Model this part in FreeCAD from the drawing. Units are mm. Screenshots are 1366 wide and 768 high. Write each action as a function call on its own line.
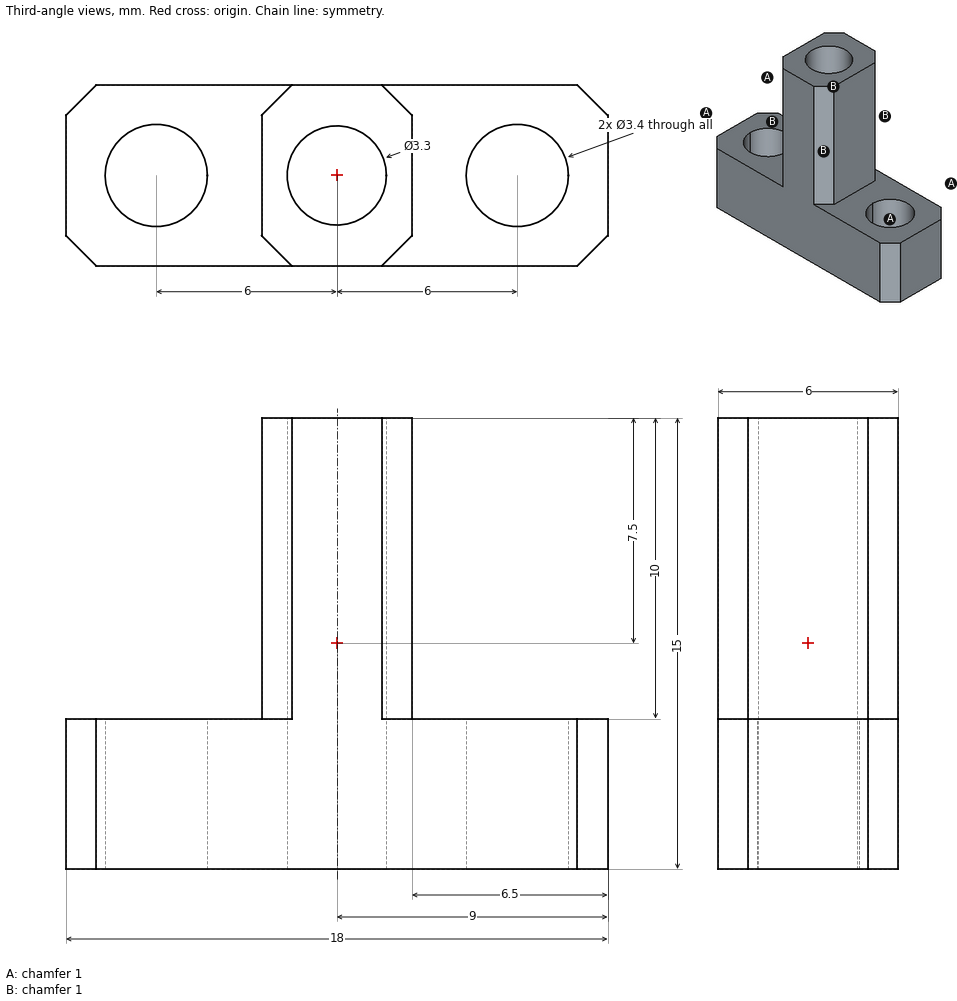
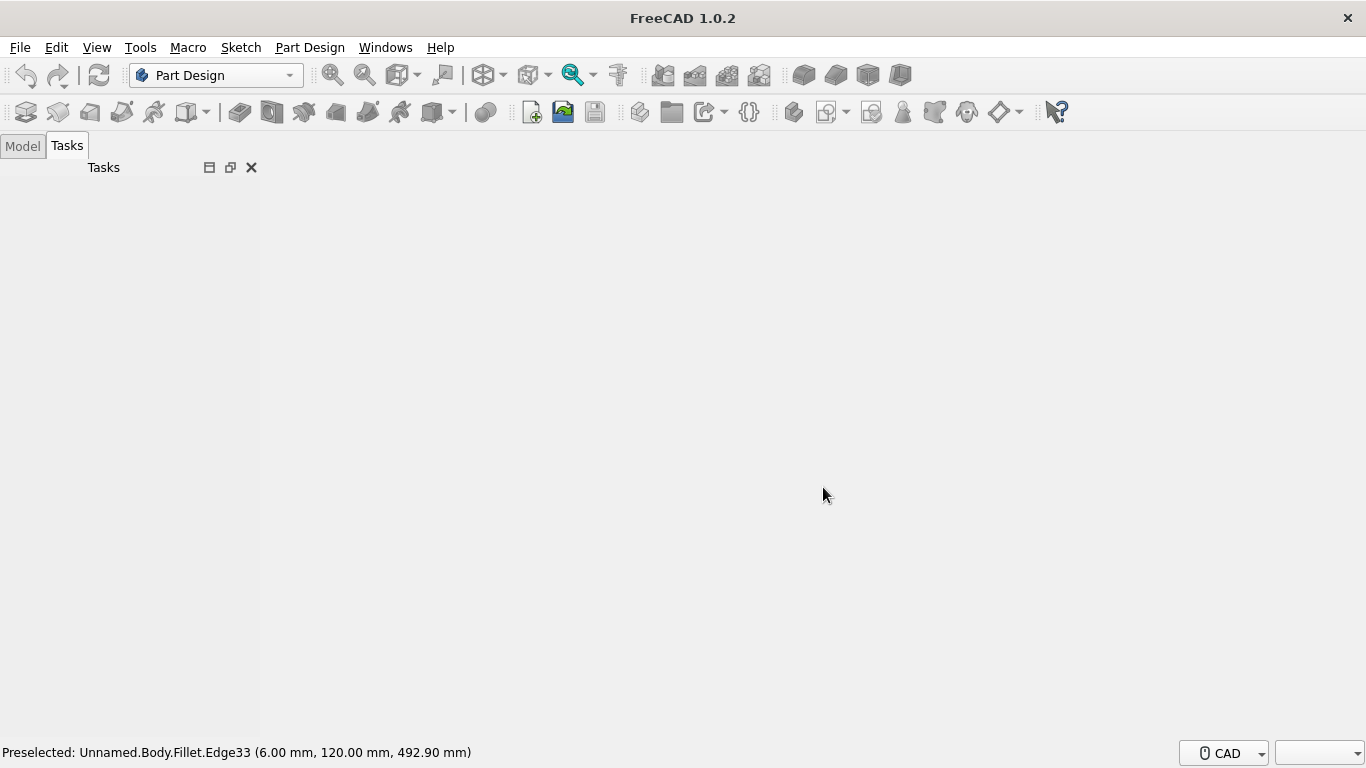
click(532, 112)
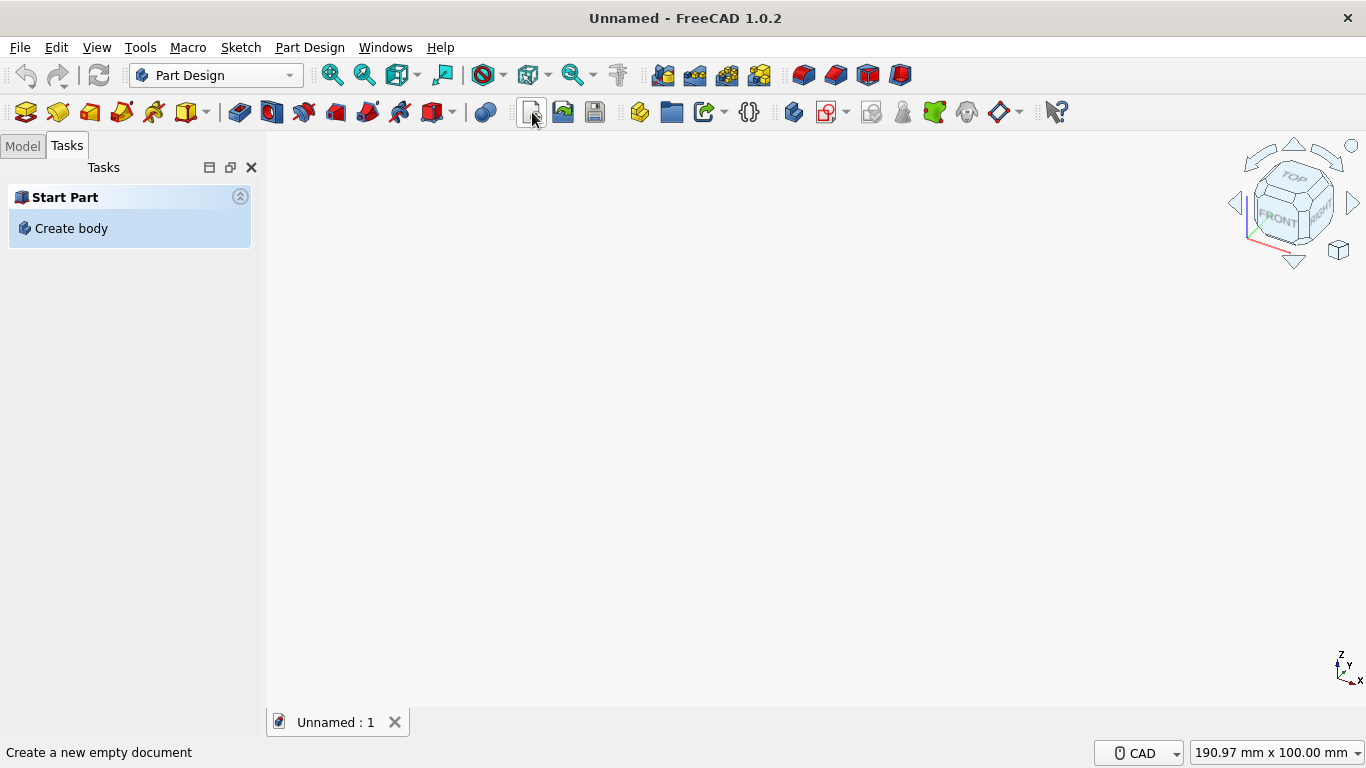
click(826, 112)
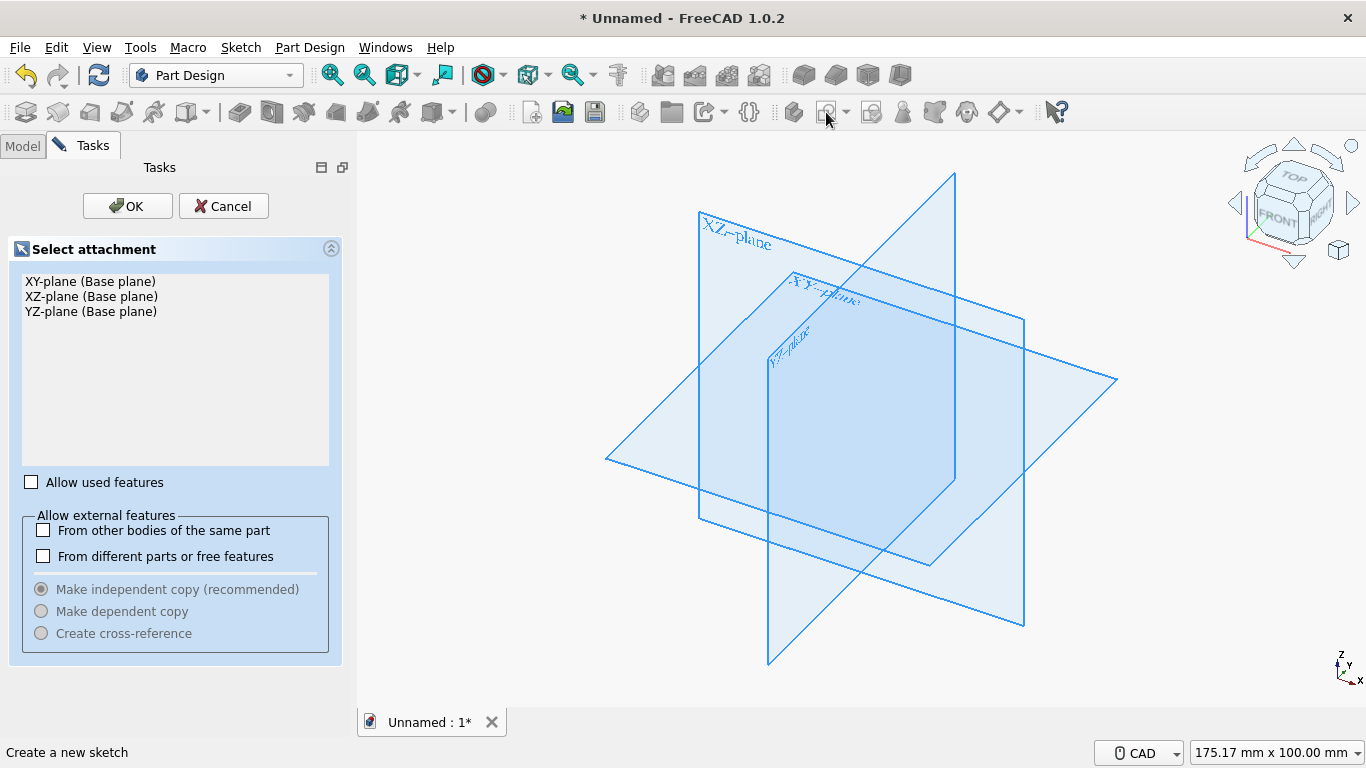
click(82, 296)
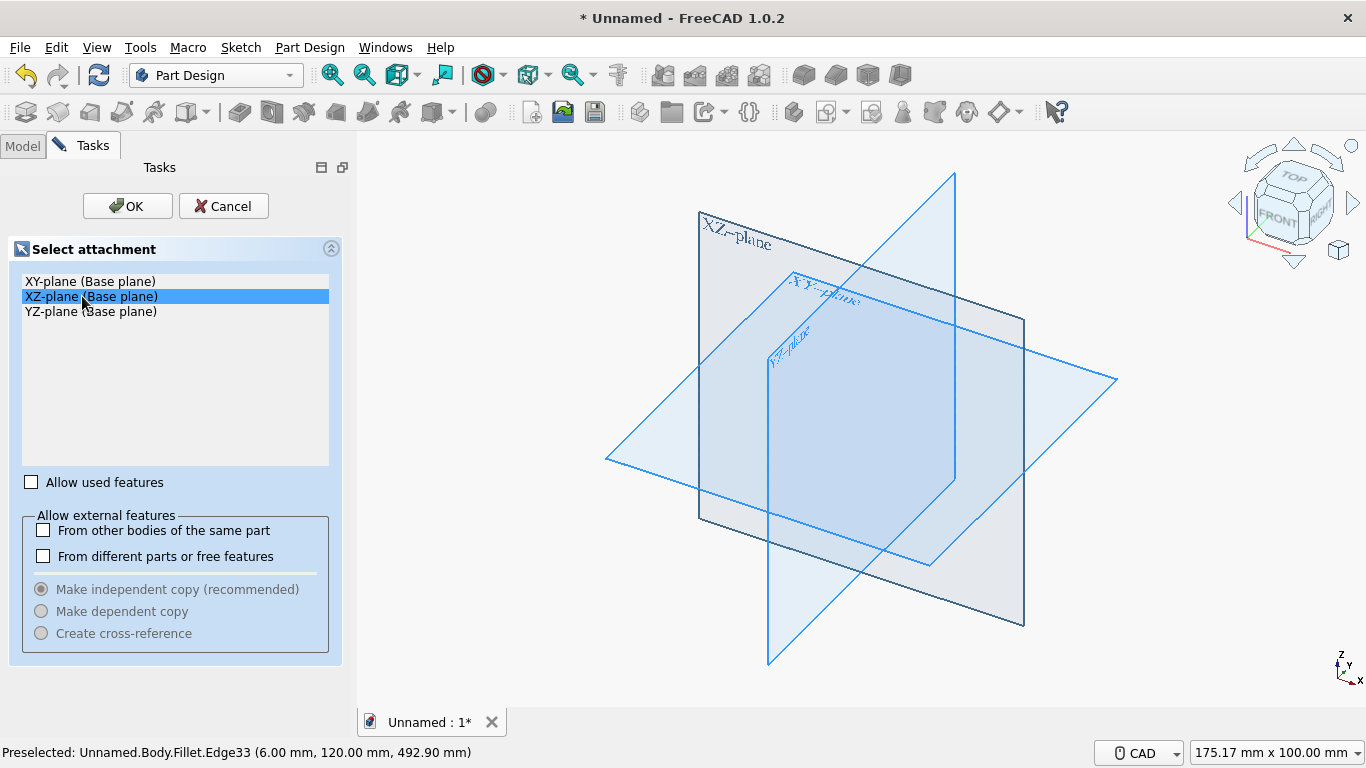
click(128, 206)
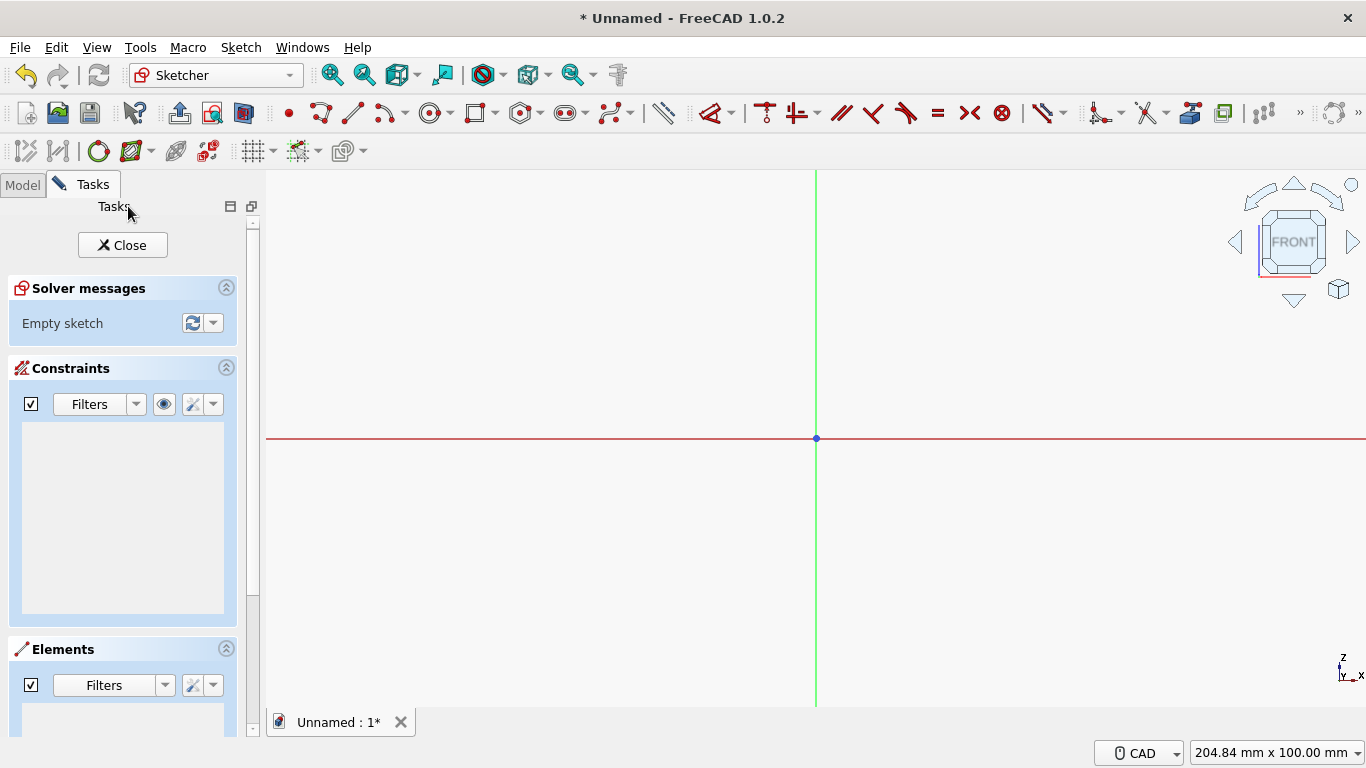
scroll(838, 438, up, 7)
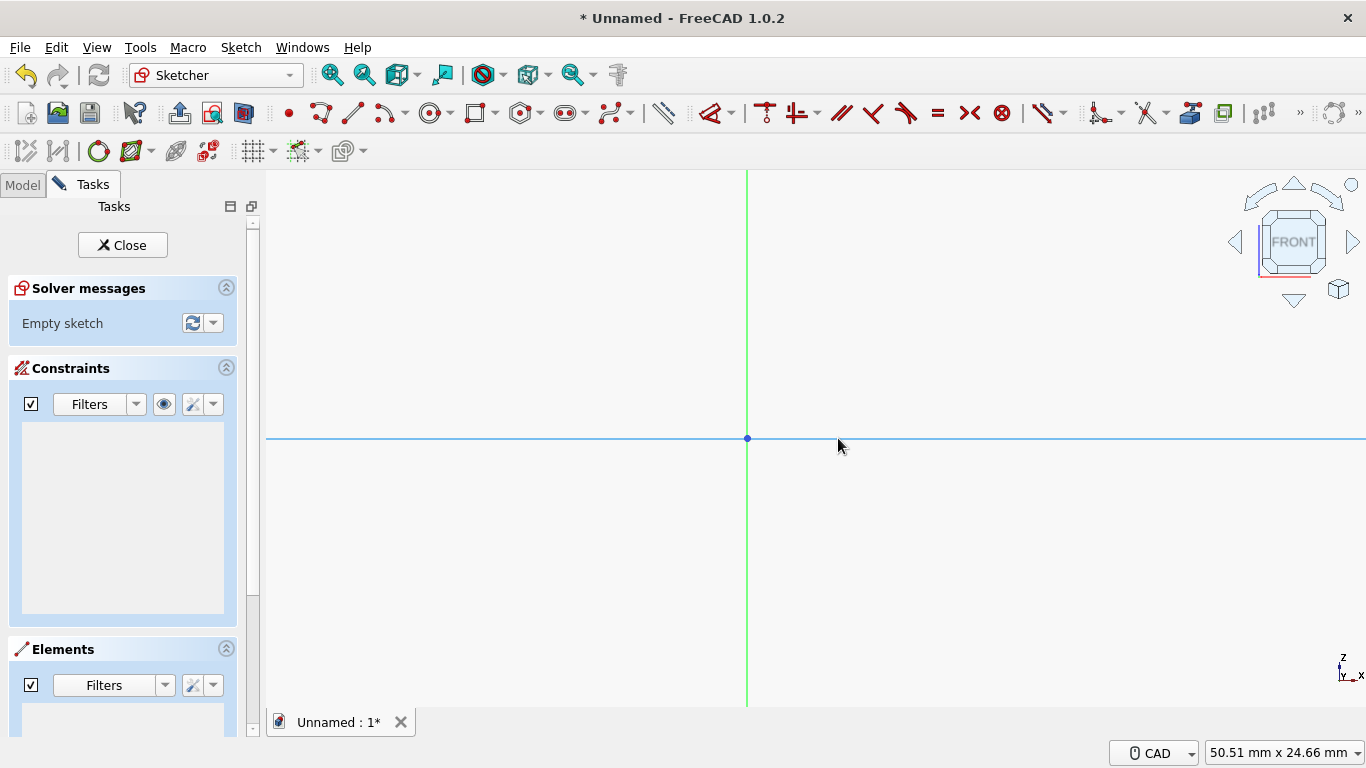
key(g)
key(v)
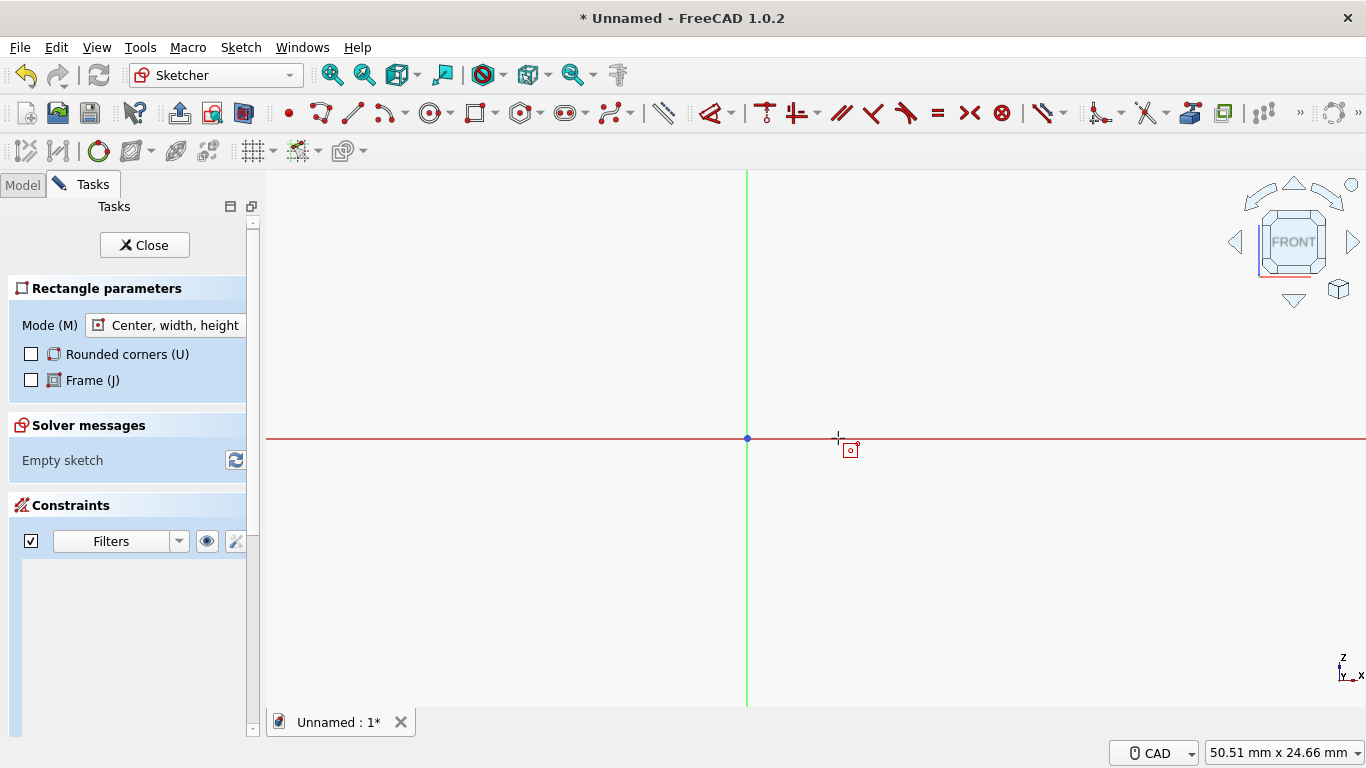
click(747, 438)
click(943, 275)
key(Escape)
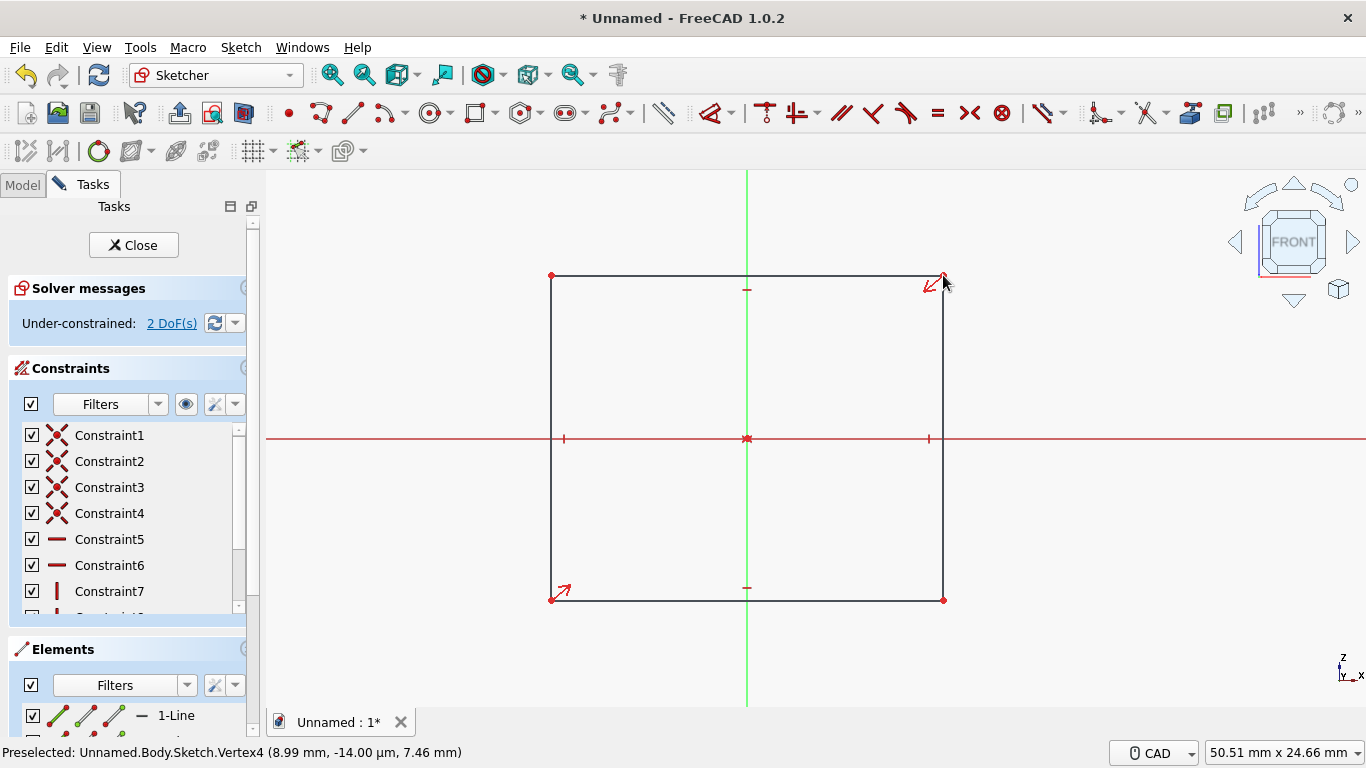
click(669, 601)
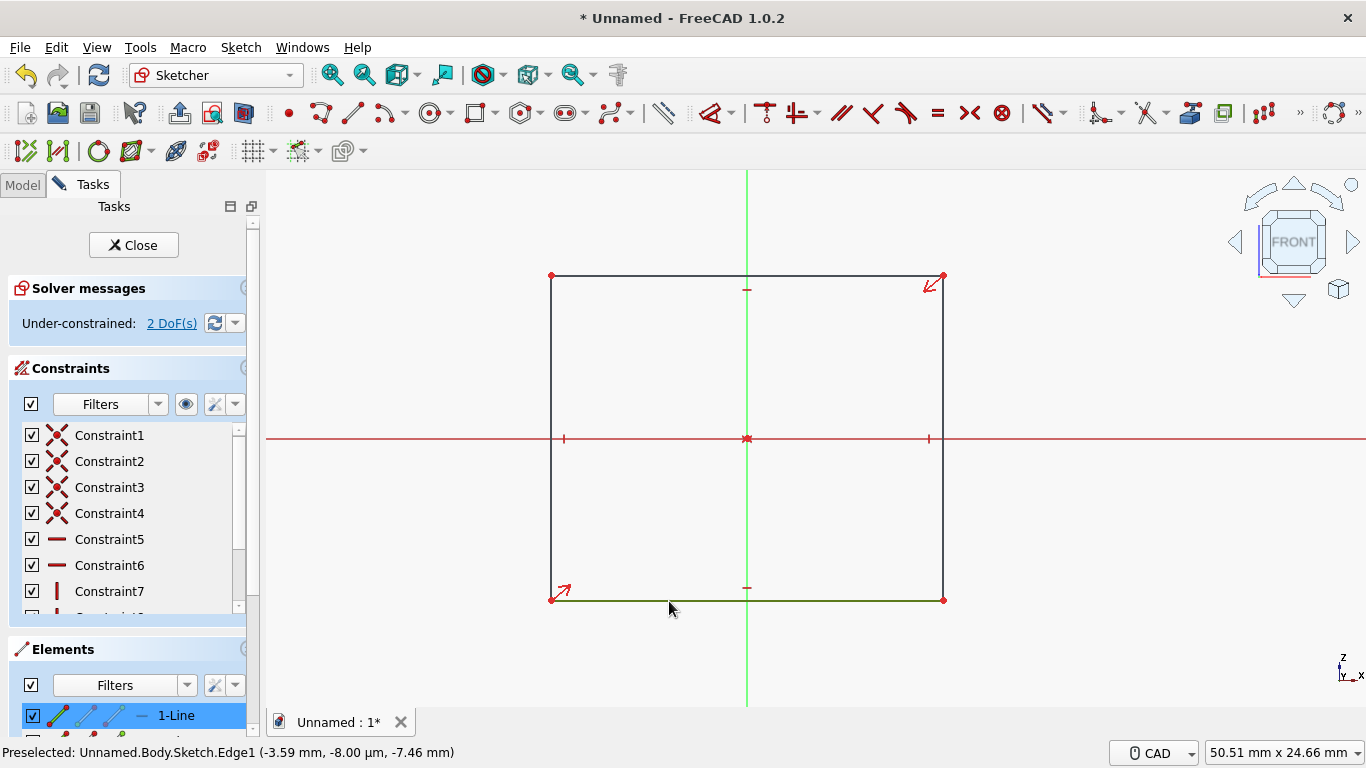
click(734, 114)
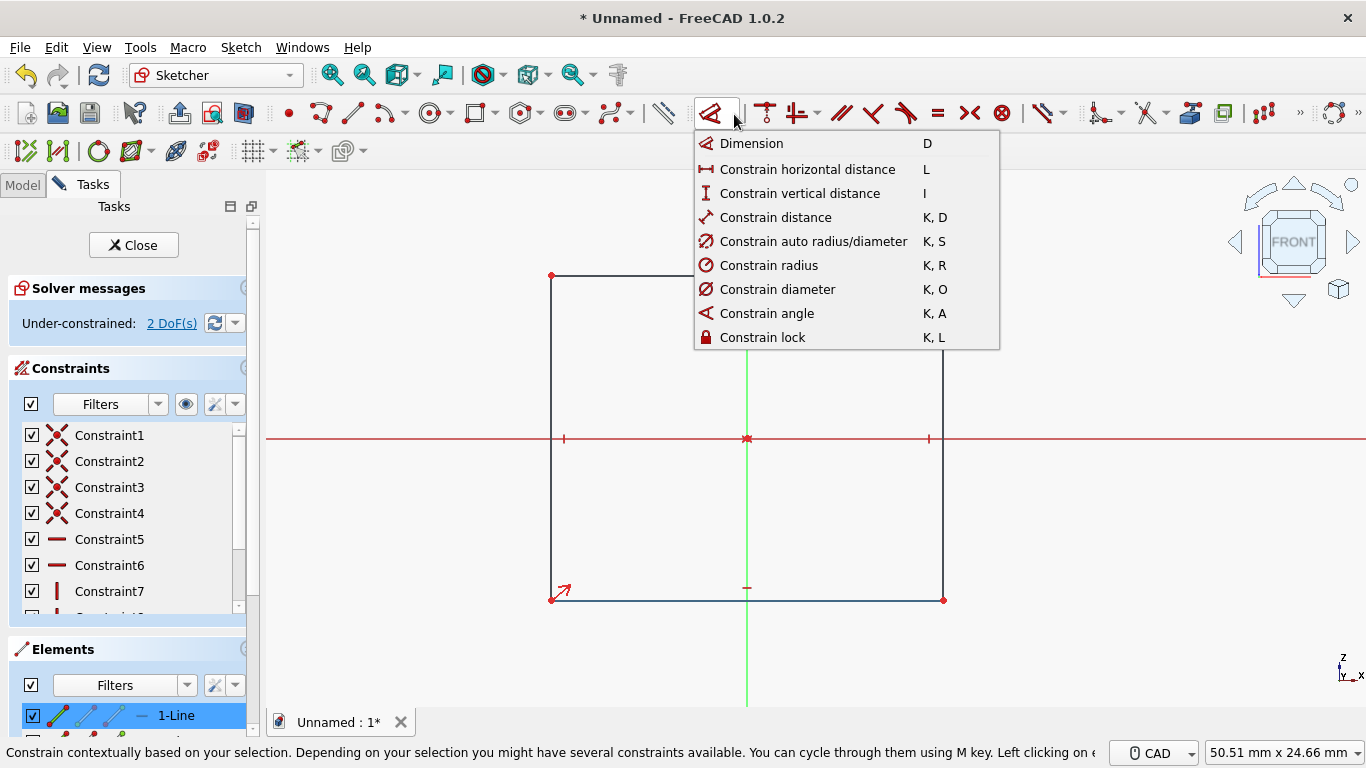
click(847, 169)